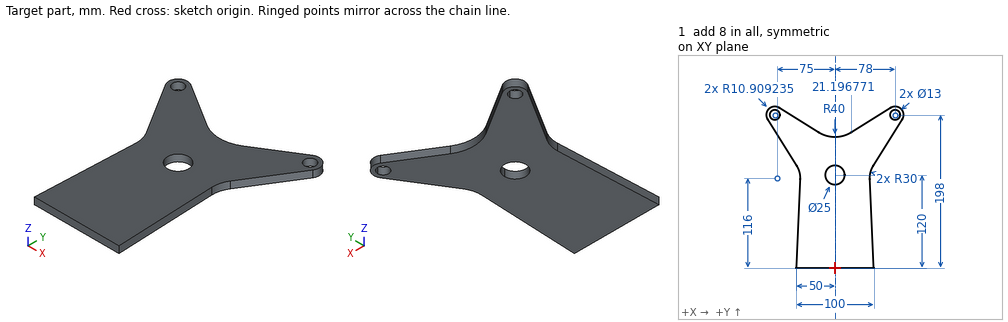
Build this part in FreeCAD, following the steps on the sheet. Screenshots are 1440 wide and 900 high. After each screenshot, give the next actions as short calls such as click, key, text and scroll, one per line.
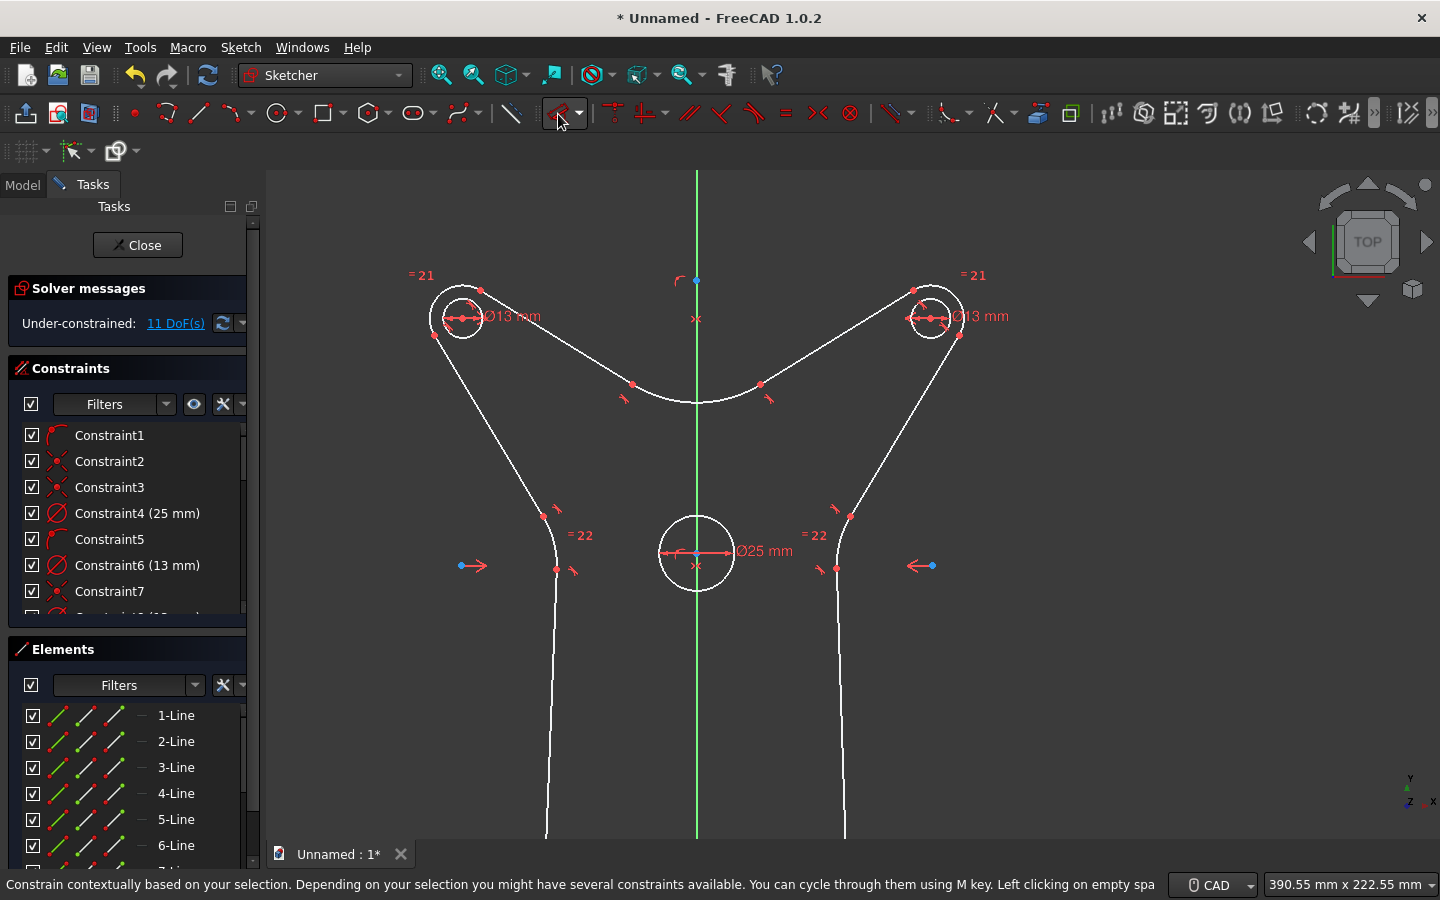
click(963, 310)
click(994, 302)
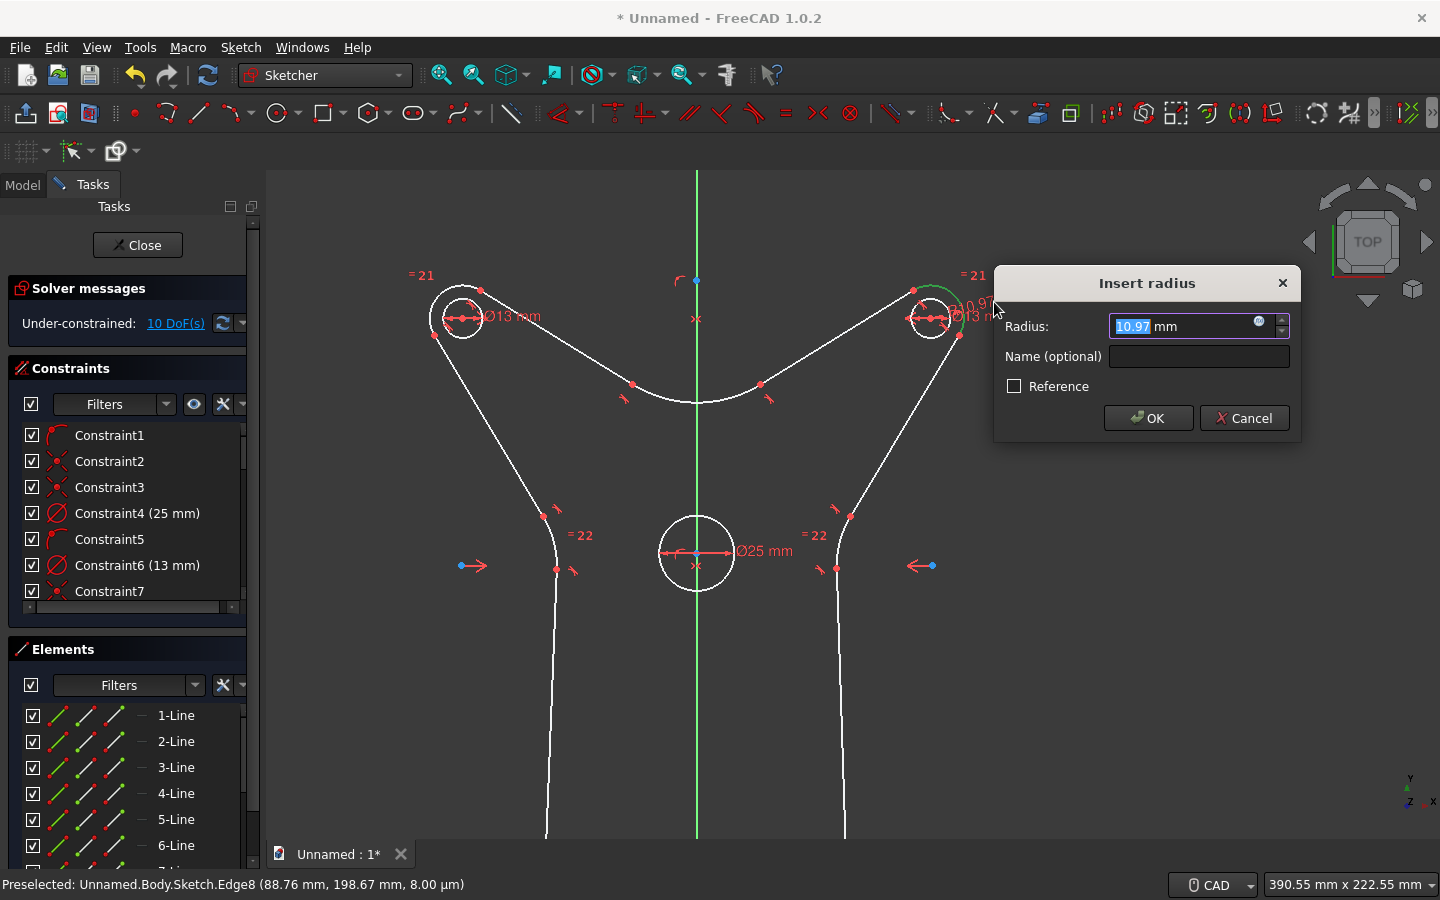
text(10.909235)
key(Return)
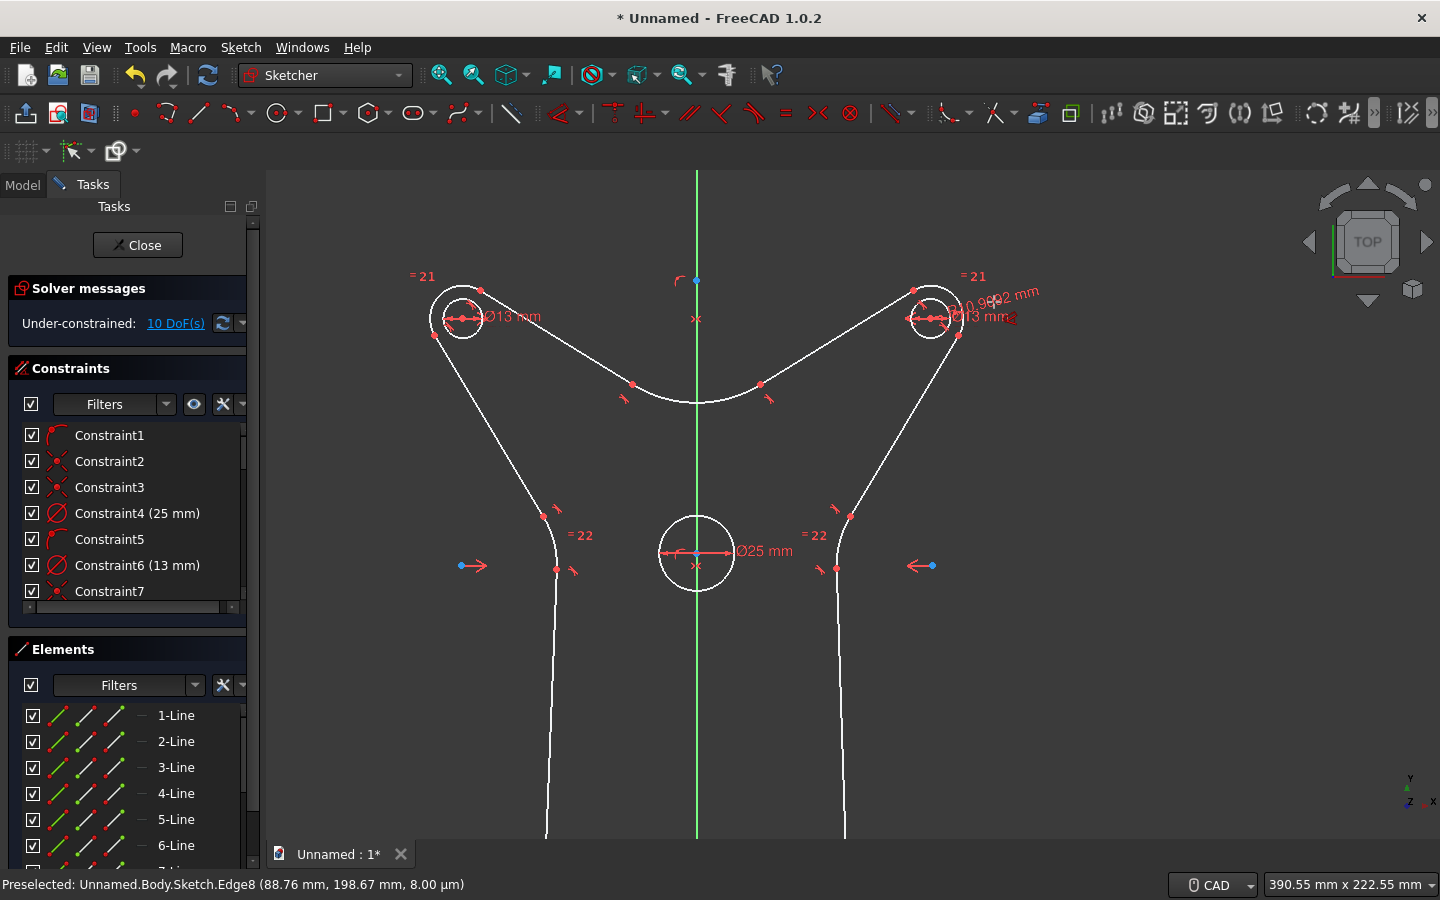
click(670, 400)
click(663, 431)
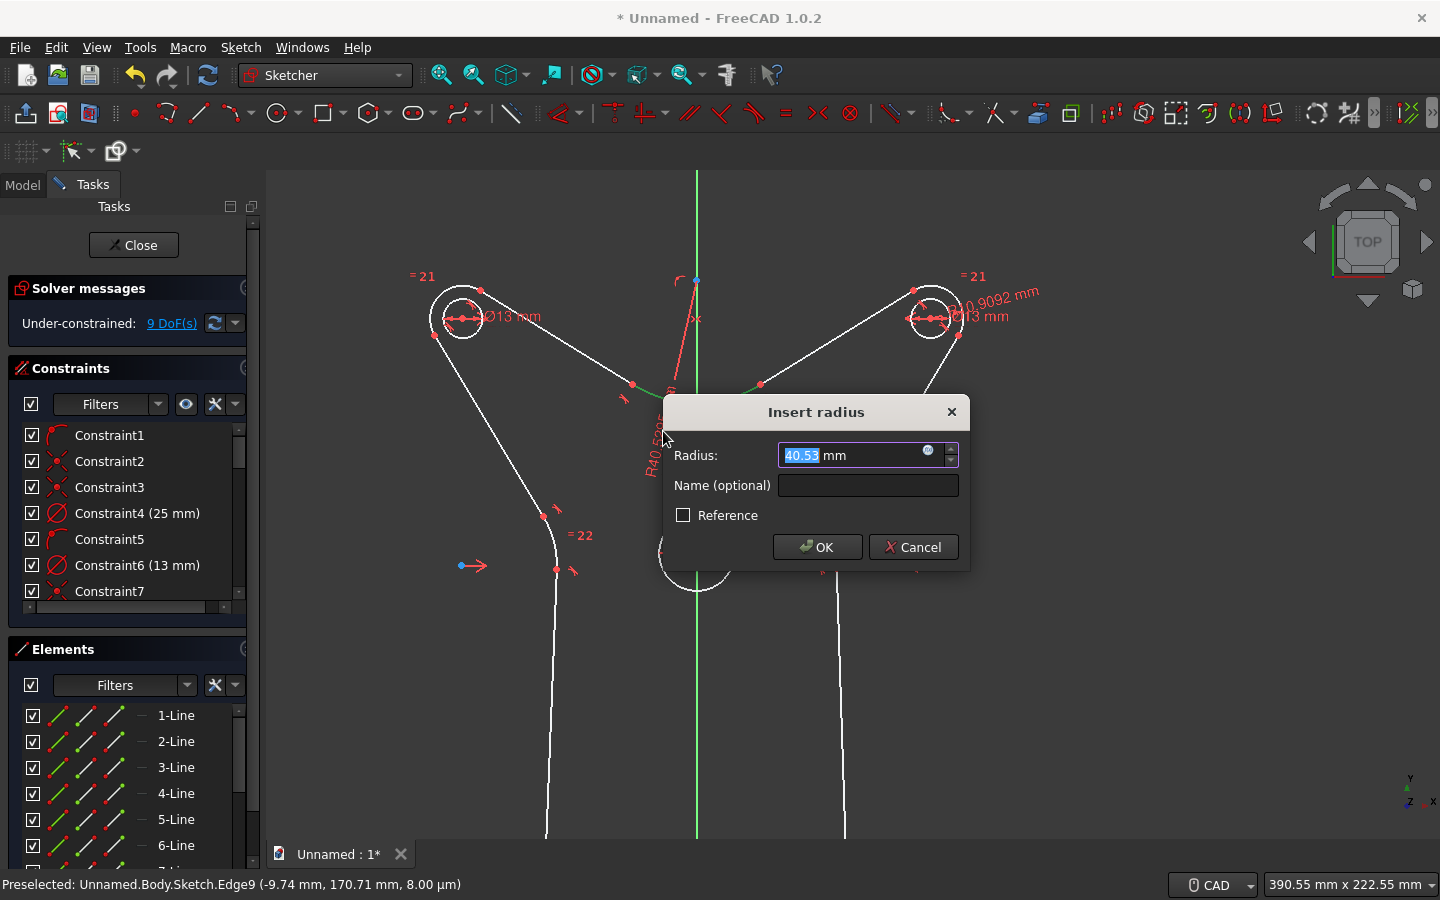
text(40)
key(Return)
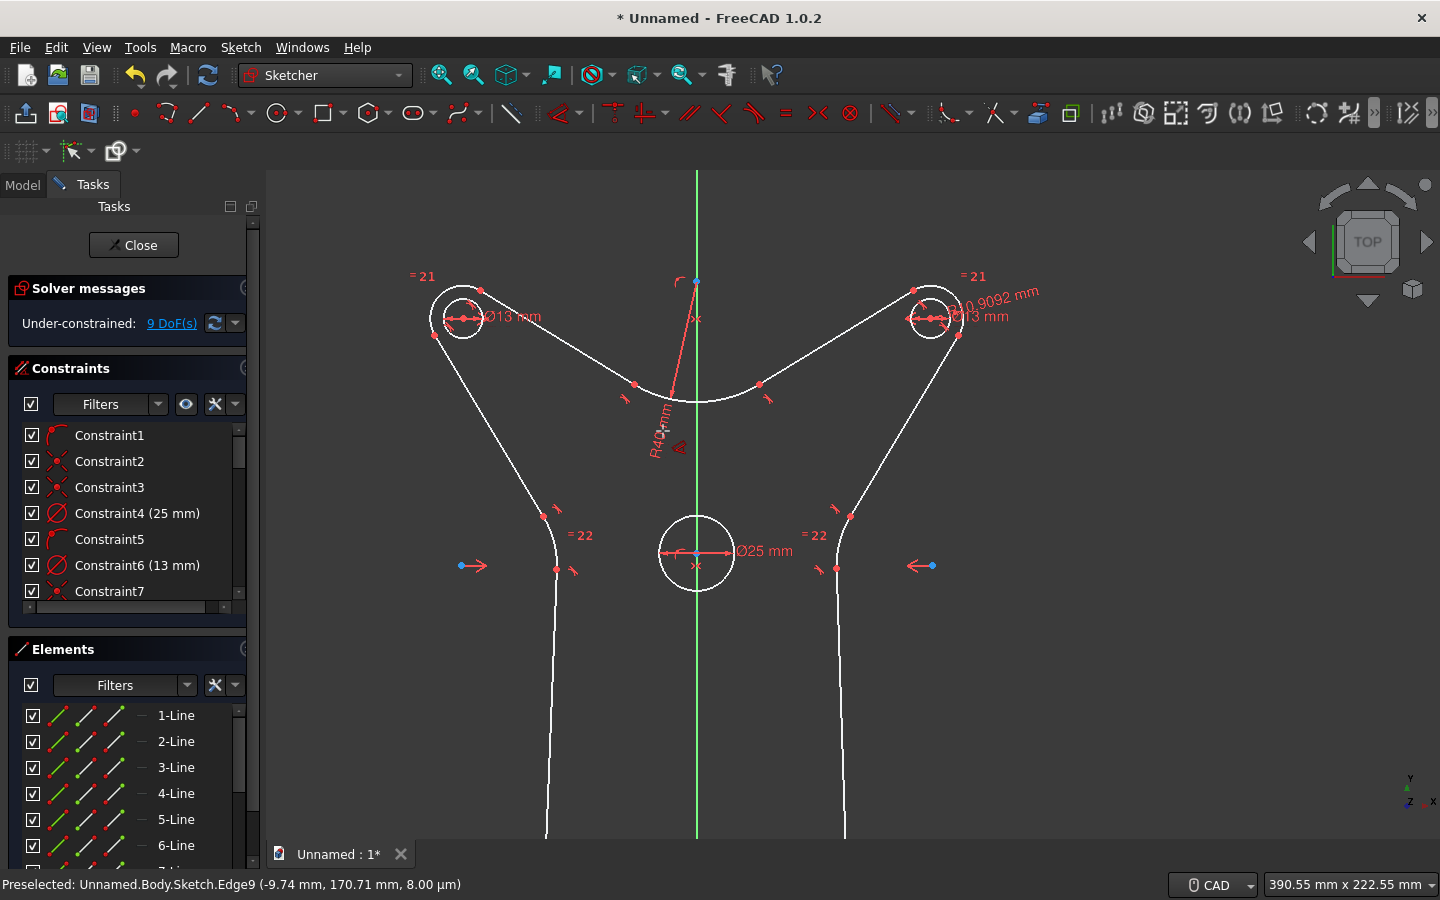
click(556, 553)
click(588, 549)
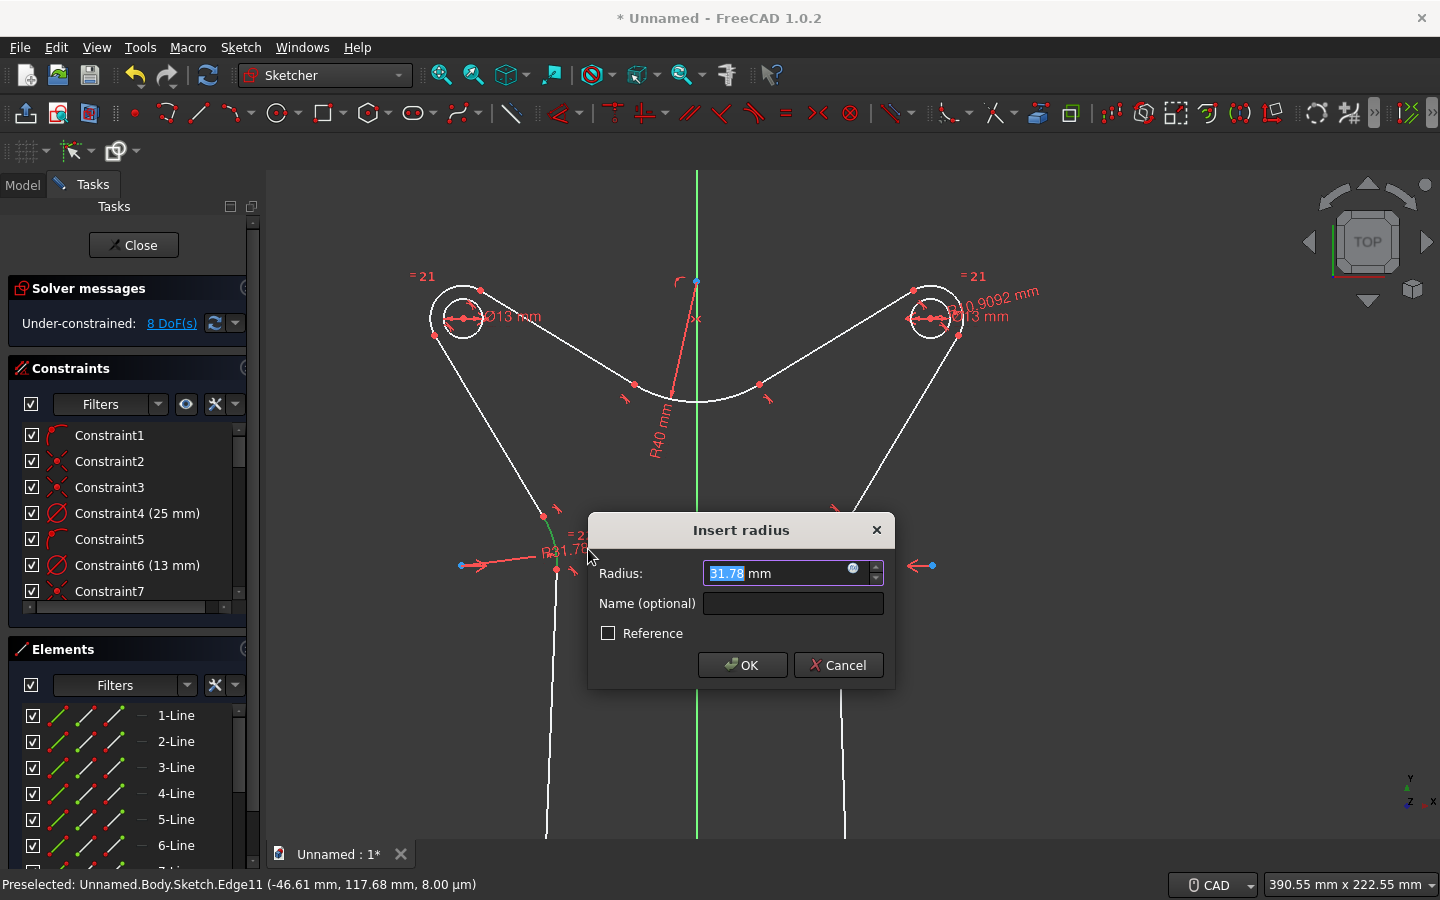
text(30)
key(Return)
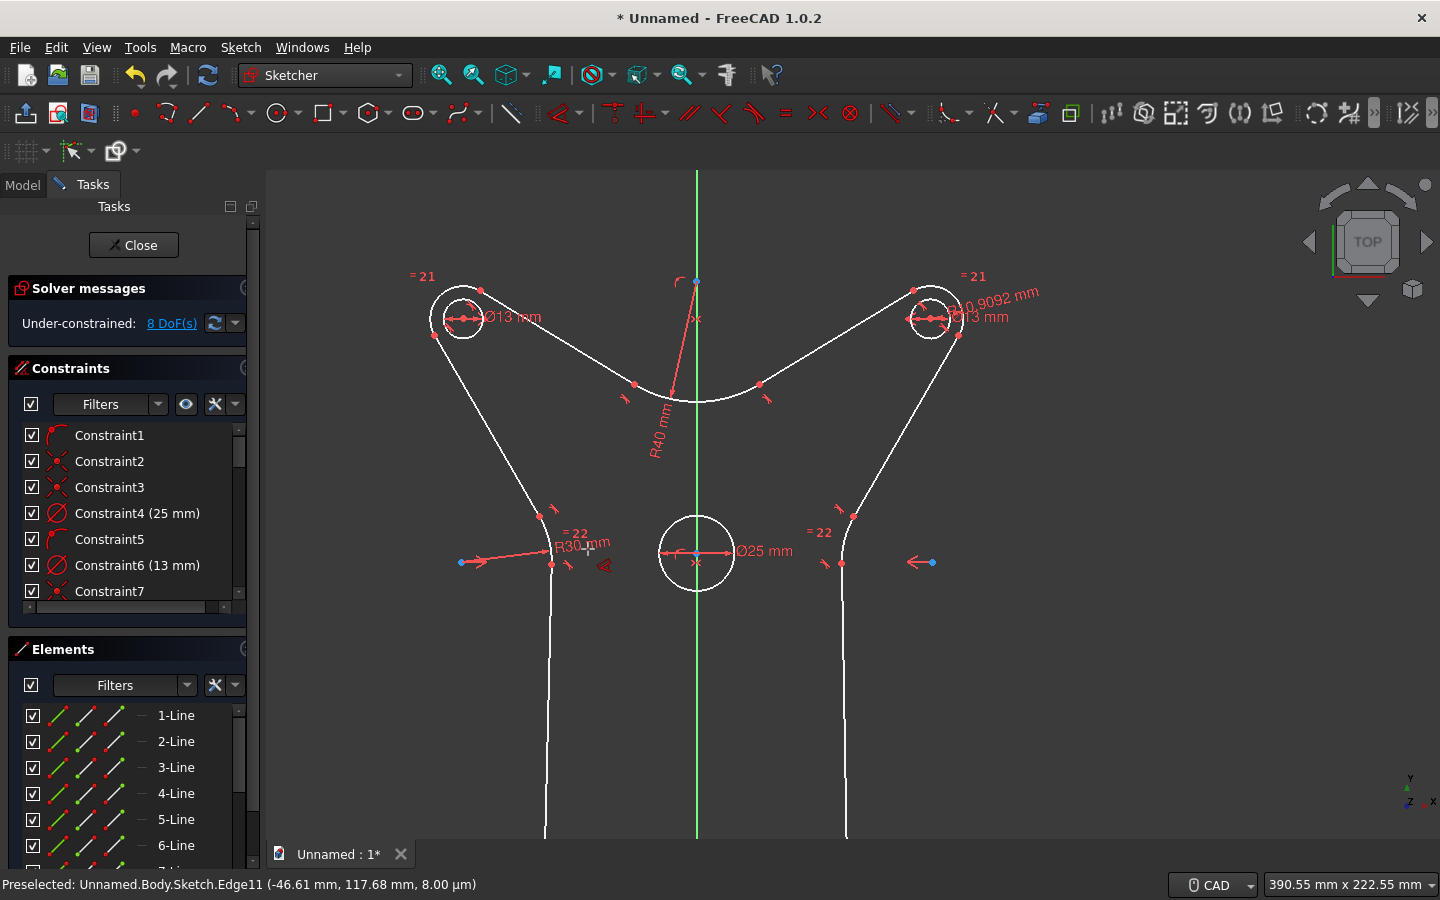
click(930, 319)
click(814, 285)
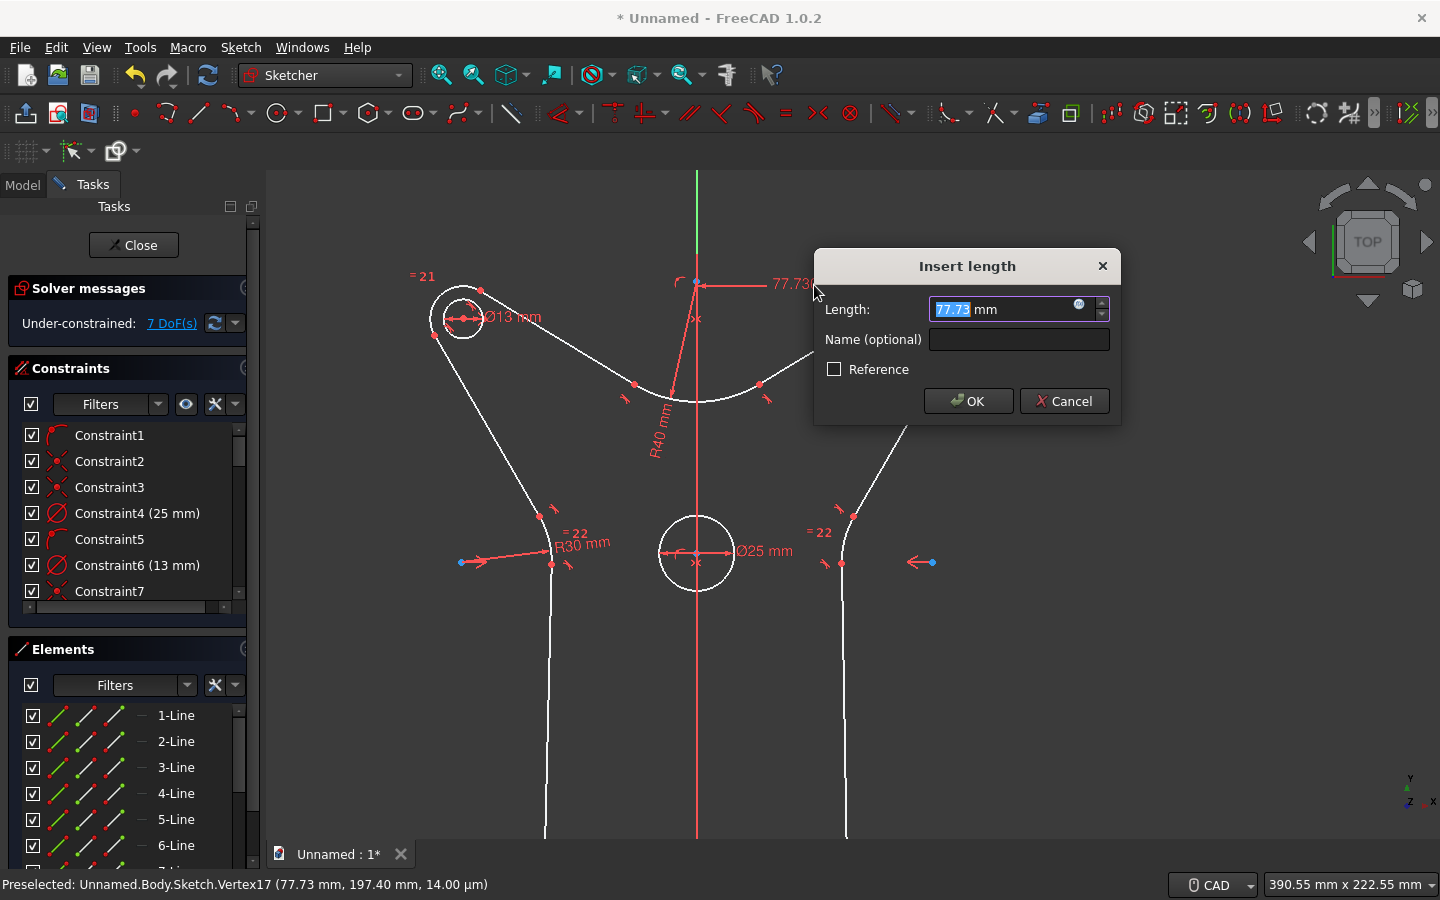
text(78)
key(Return)